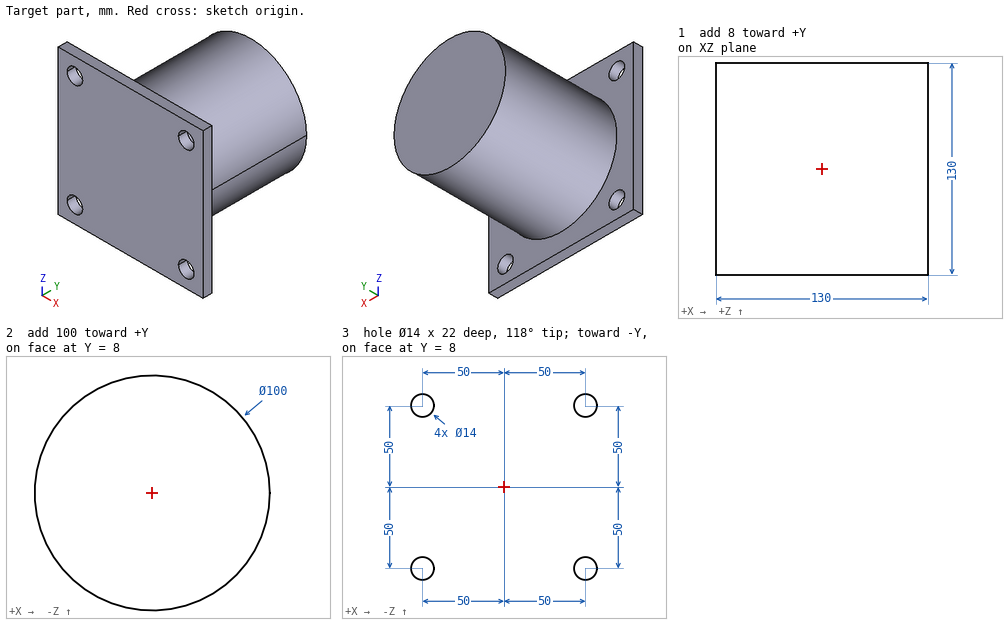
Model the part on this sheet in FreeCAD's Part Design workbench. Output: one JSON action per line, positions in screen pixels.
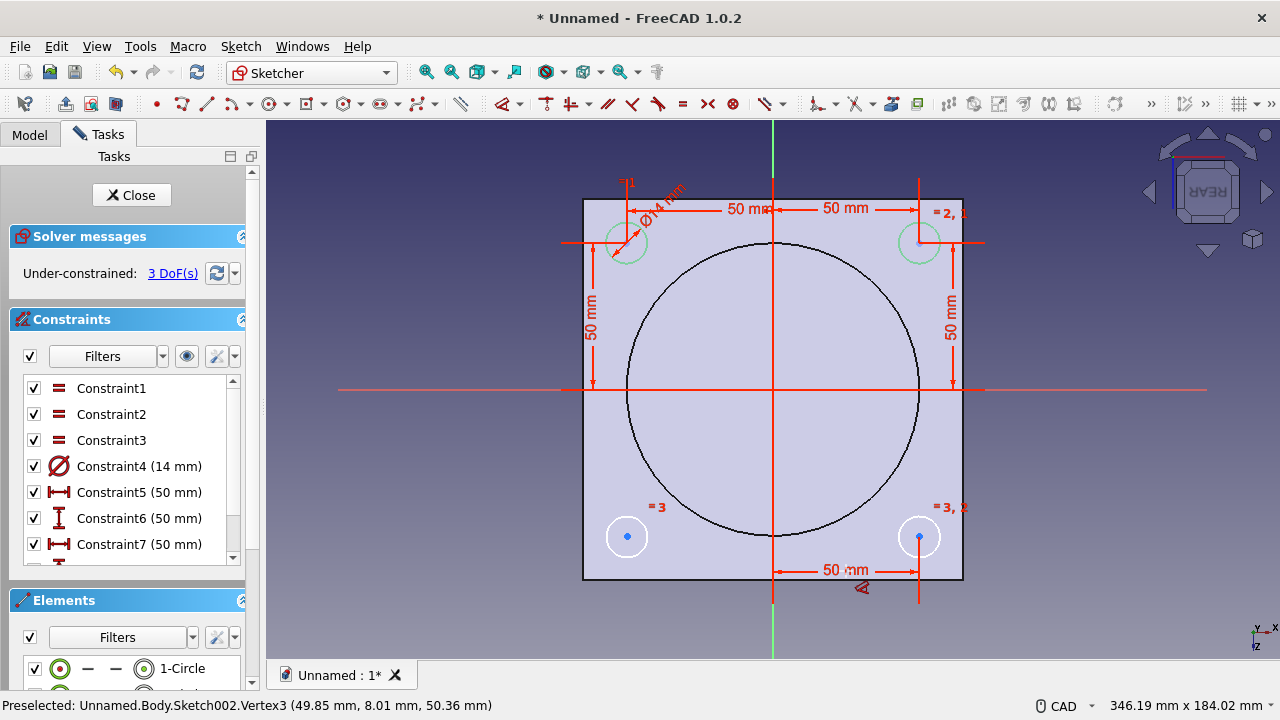
{"action": "left_click", "coordinate": [919, 537]}
{"action": "left_click", "coordinate": [953, 463]}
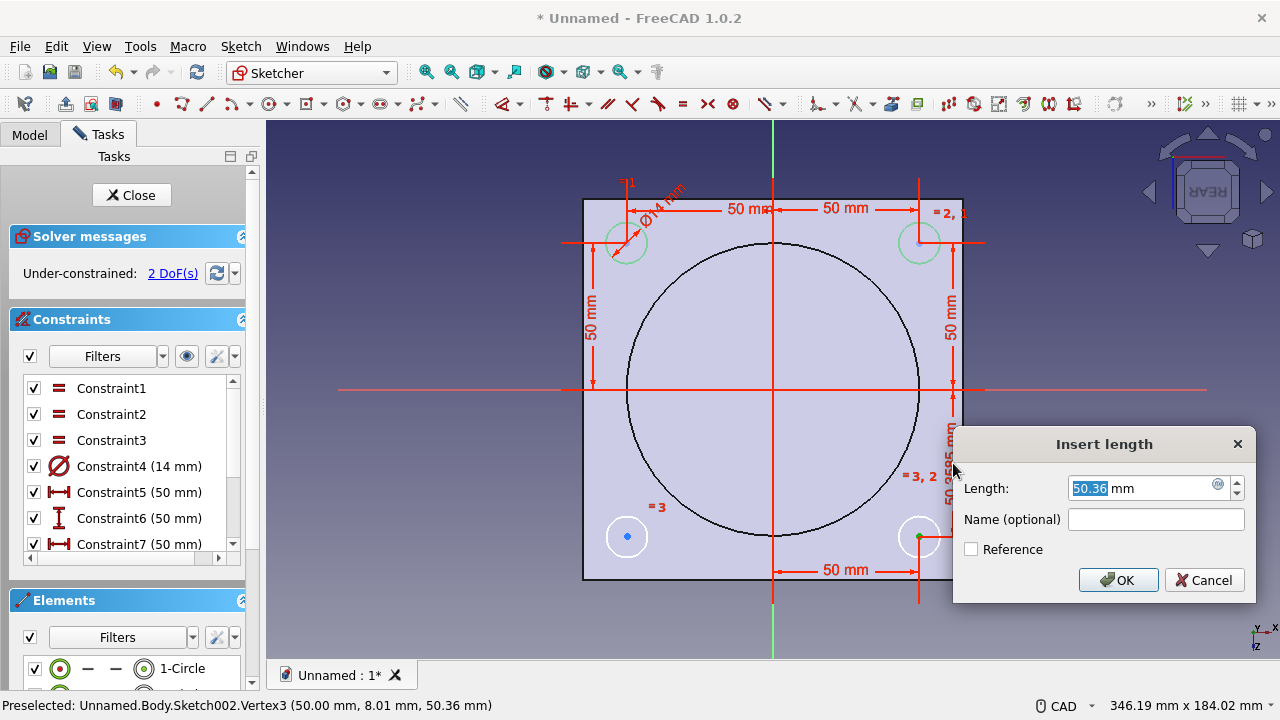
{"action": "type", "text": "50"}
{"action": "key", "text": "Return"}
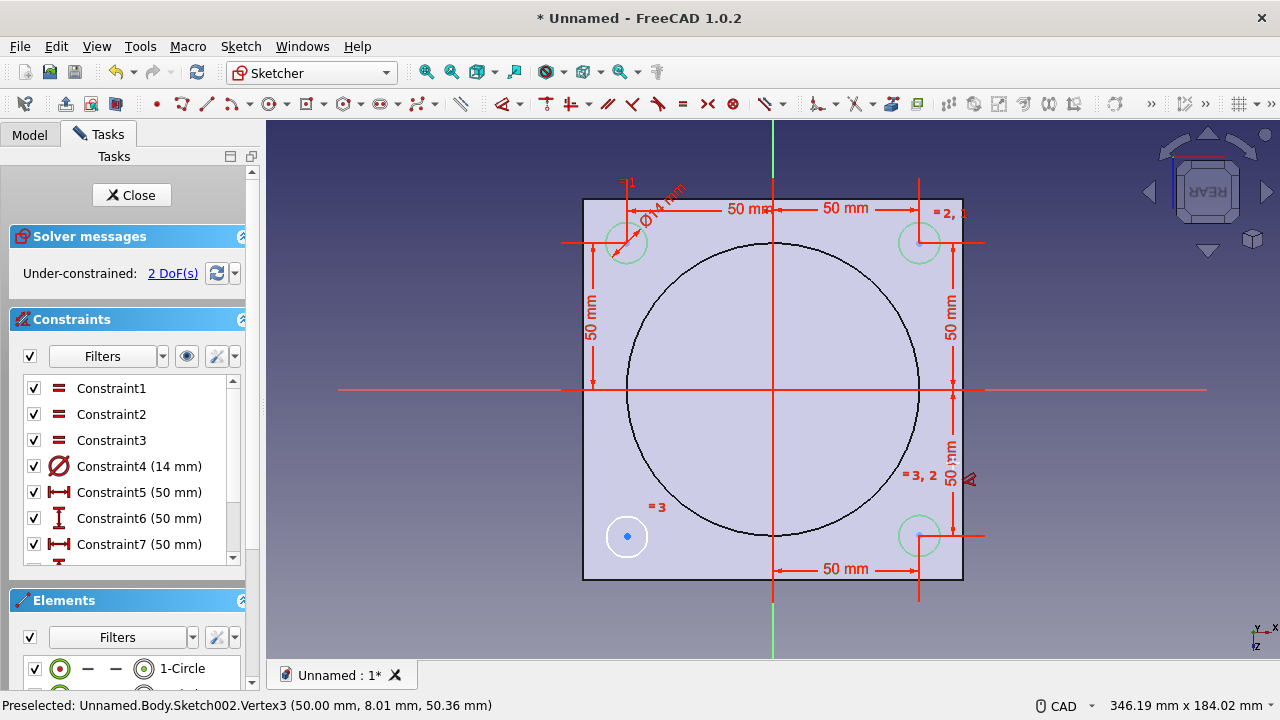
{"action": "left_click", "coordinate": [627, 537]}
{"action": "left_click", "coordinate": [700, 571]}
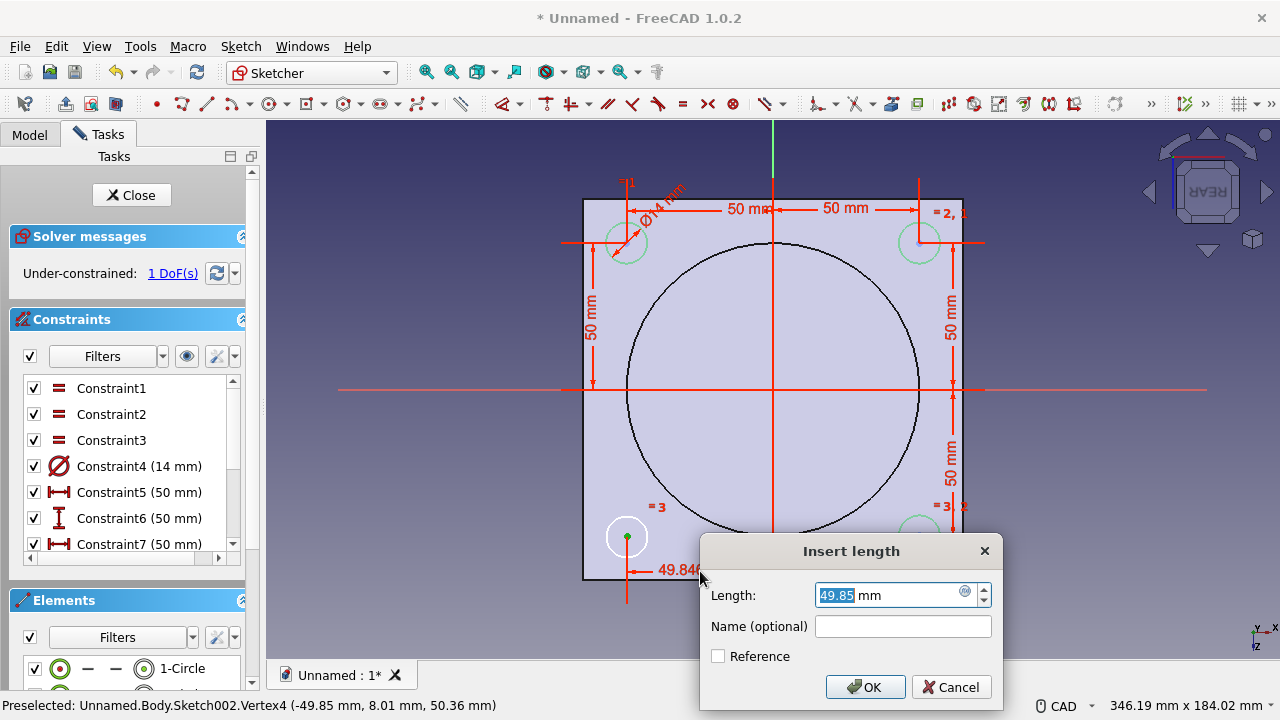
{"action": "type", "text": "50"}
{"action": "key", "text": "Return"}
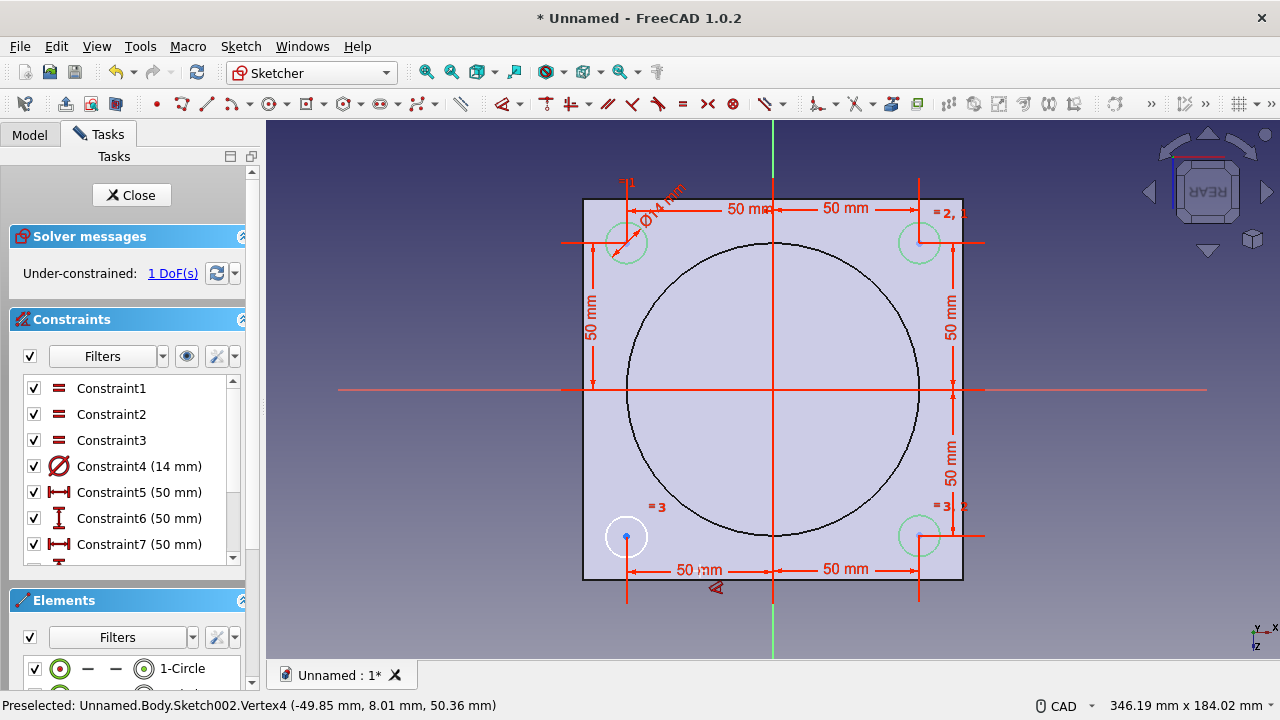
{"action": "left_click", "coordinate": [627, 537]}
{"action": "left_click", "coordinate": [593, 463]}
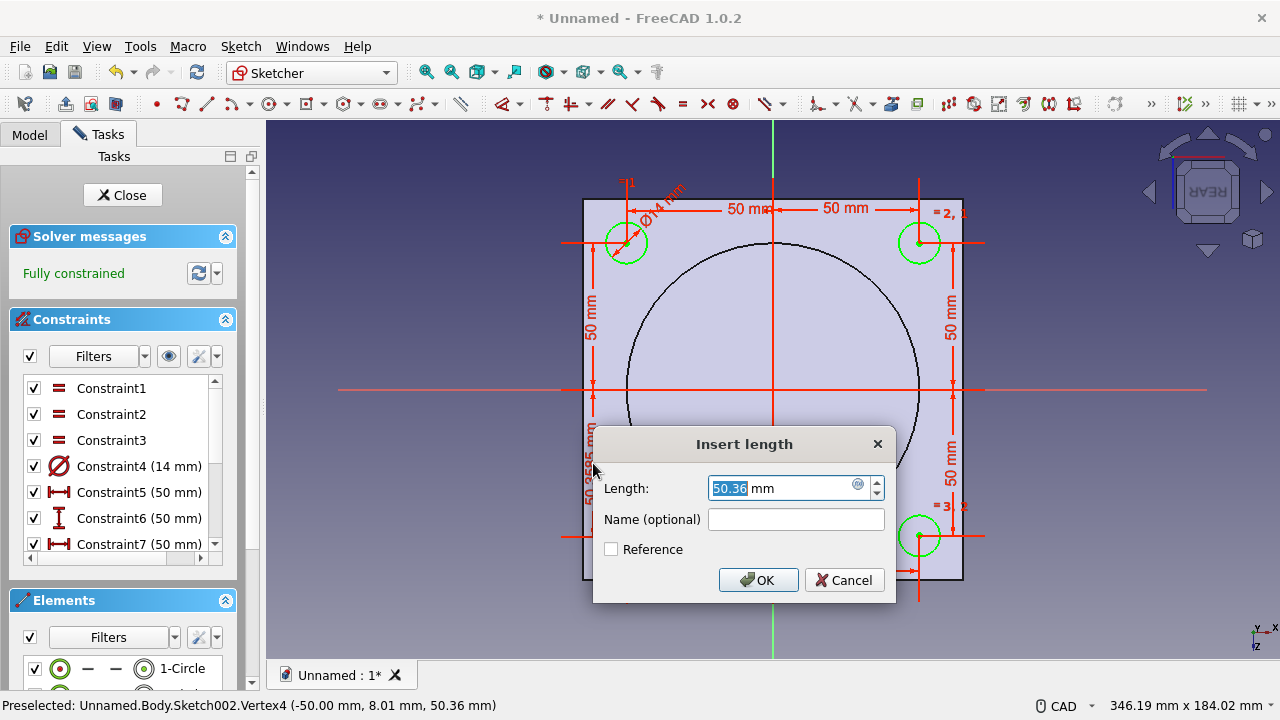
{"action": "type", "text": "50"}
{"action": "key", "text": "Return"}
{"action": "key", "text": "Escape"}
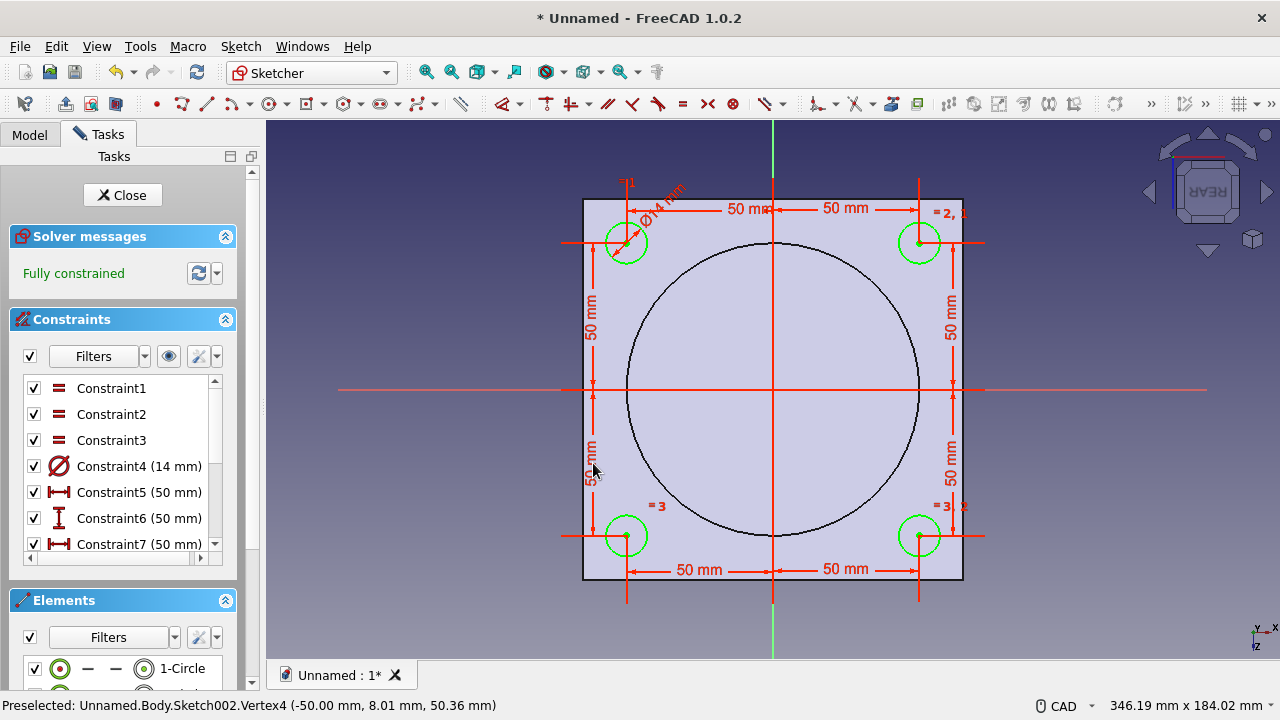
{"action": "left_click", "coordinate": [123, 195]}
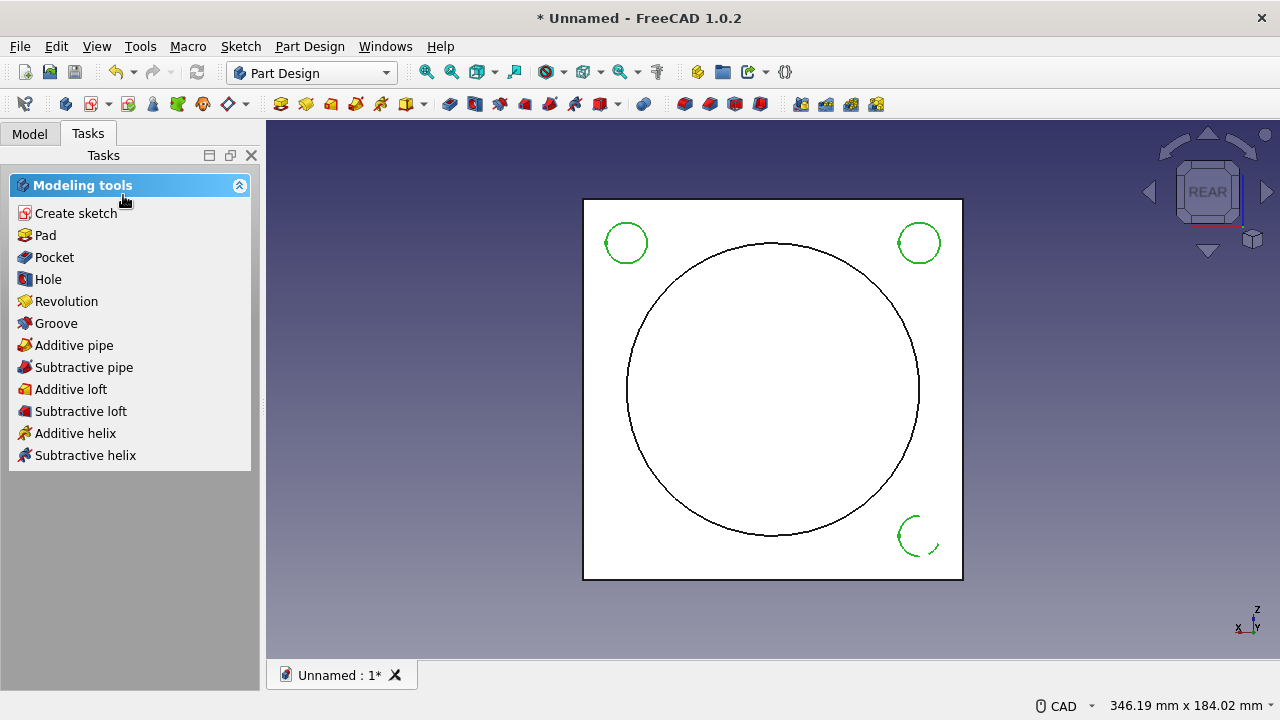
{"action": "left_click", "coordinate": [475, 104]}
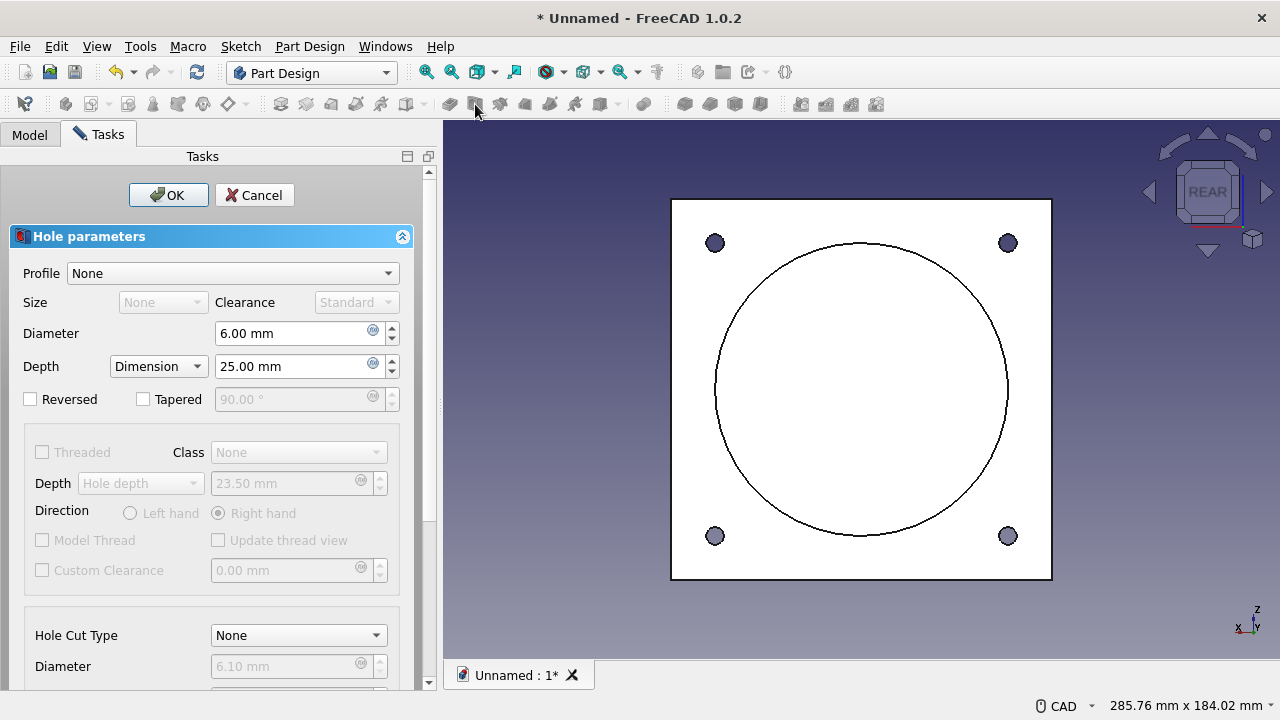
{"action": "triple_click", "coordinate": [300, 334]}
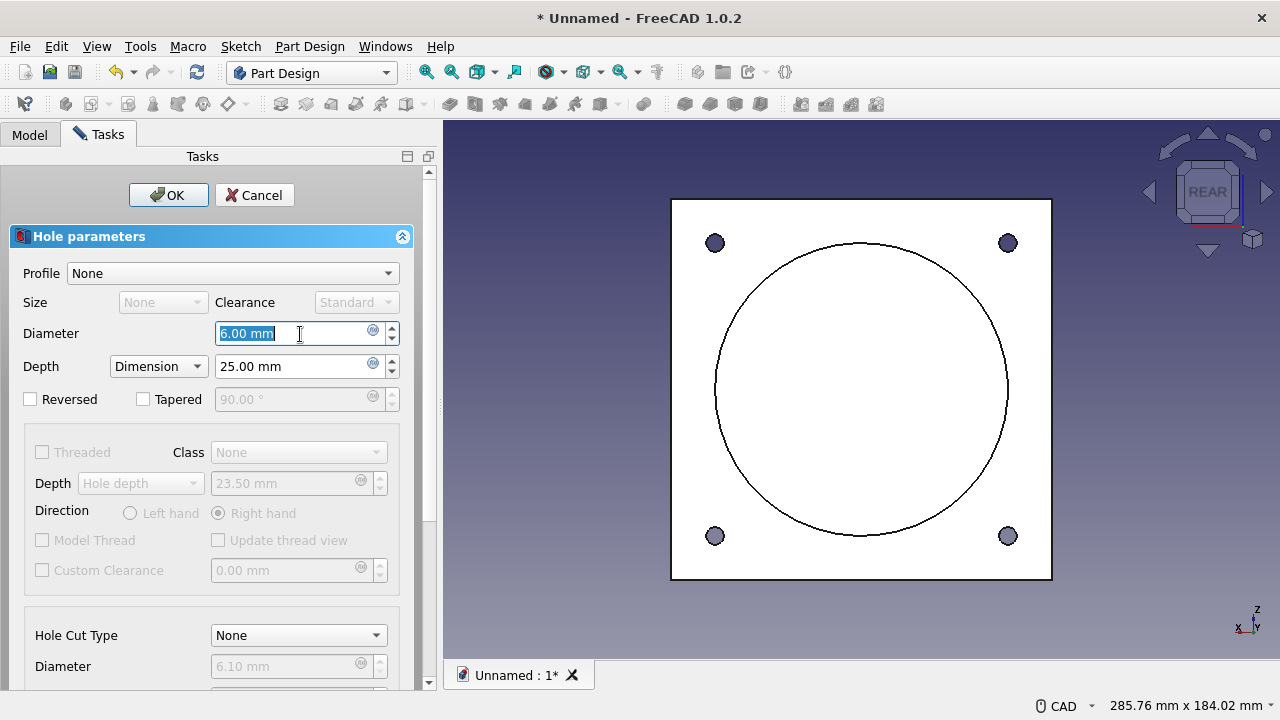
{"action": "type", "text": "14"}
{"action": "key", "text": "Tab"}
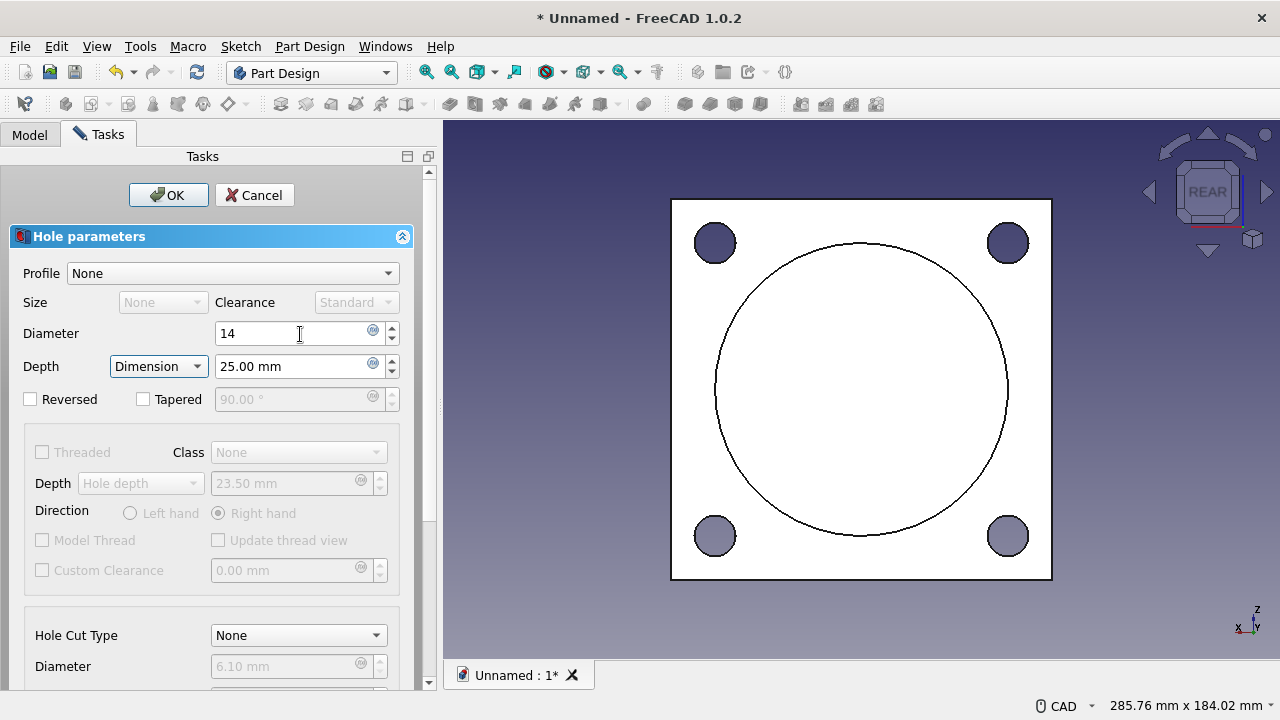
{"action": "triple_click", "coordinate": [300, 366]}